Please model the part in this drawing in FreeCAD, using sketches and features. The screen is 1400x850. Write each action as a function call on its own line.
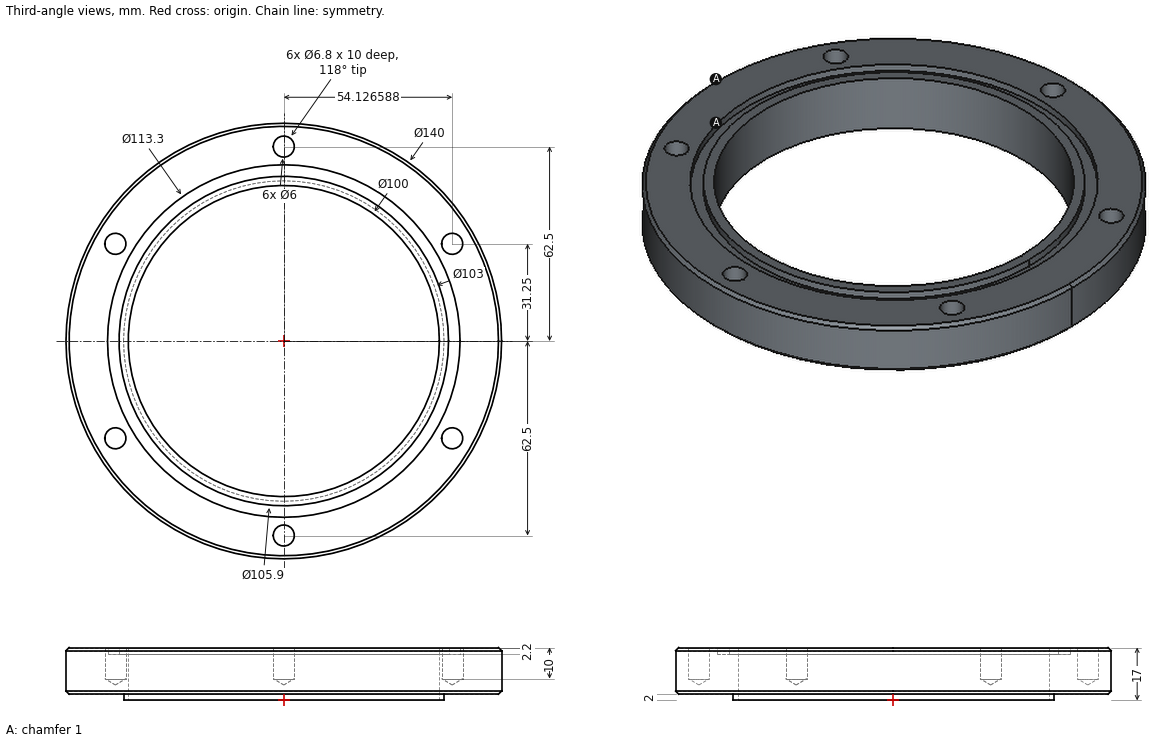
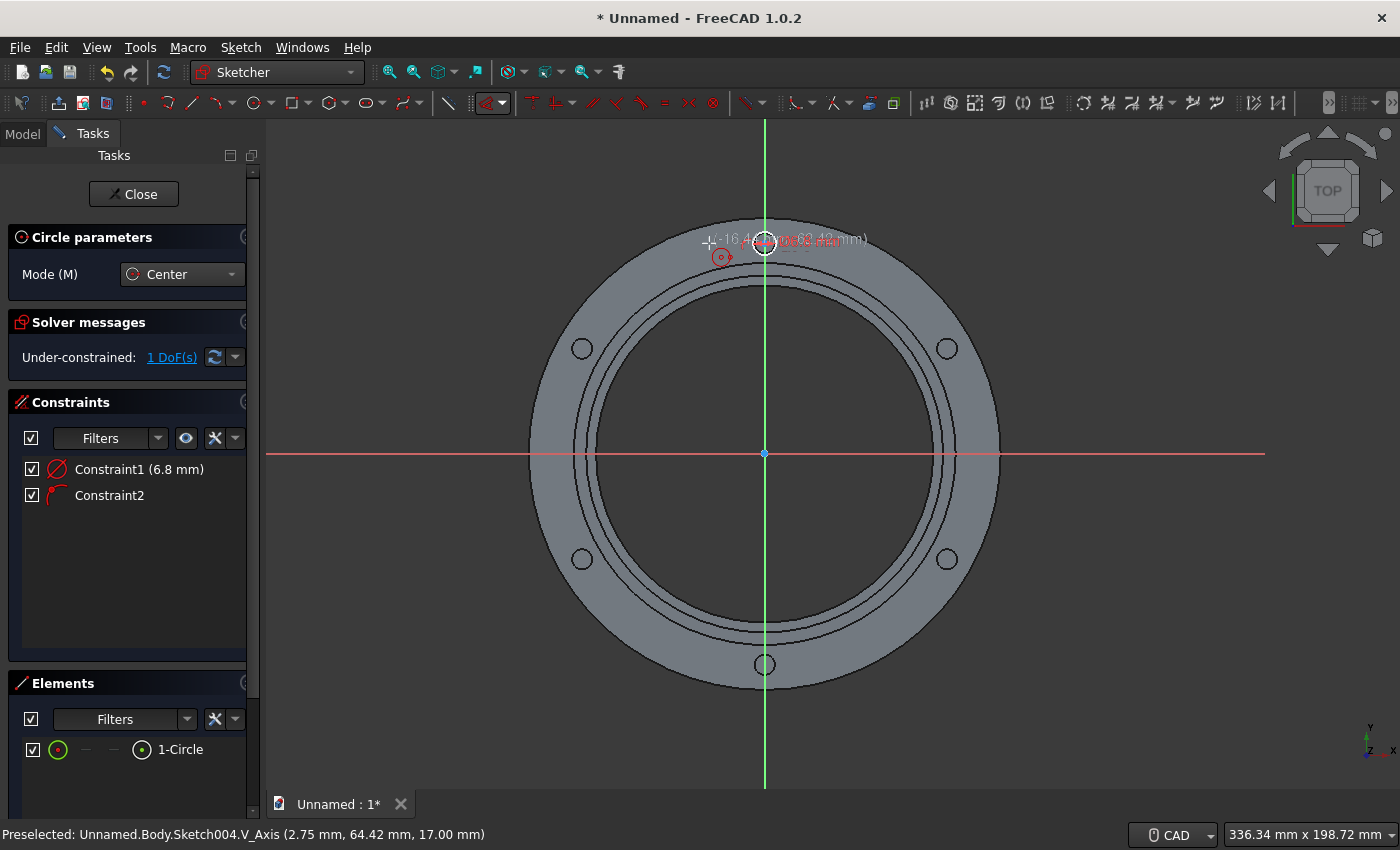
scroll(947, 349, up, 4)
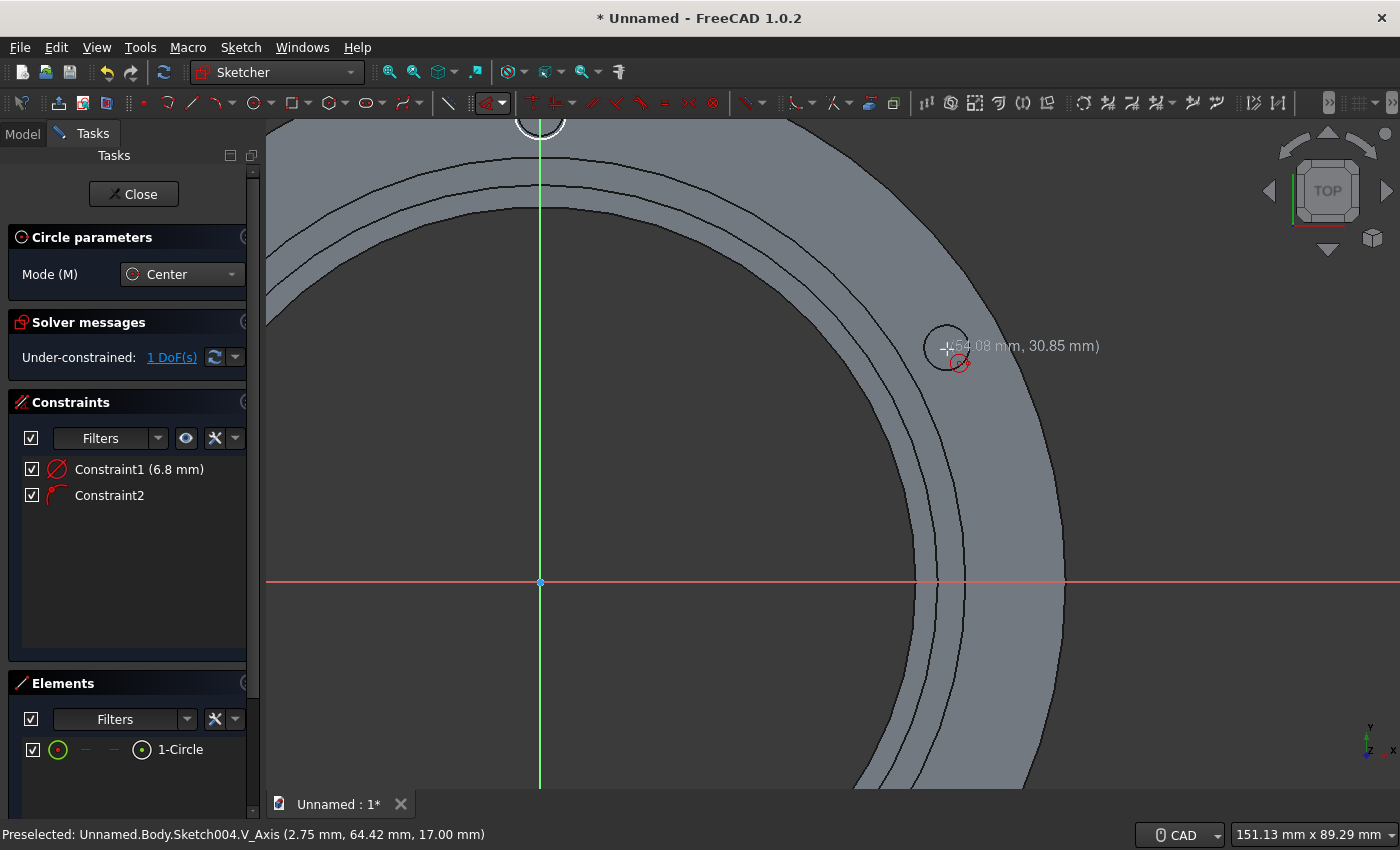
click(947, 348)
move(965, 330)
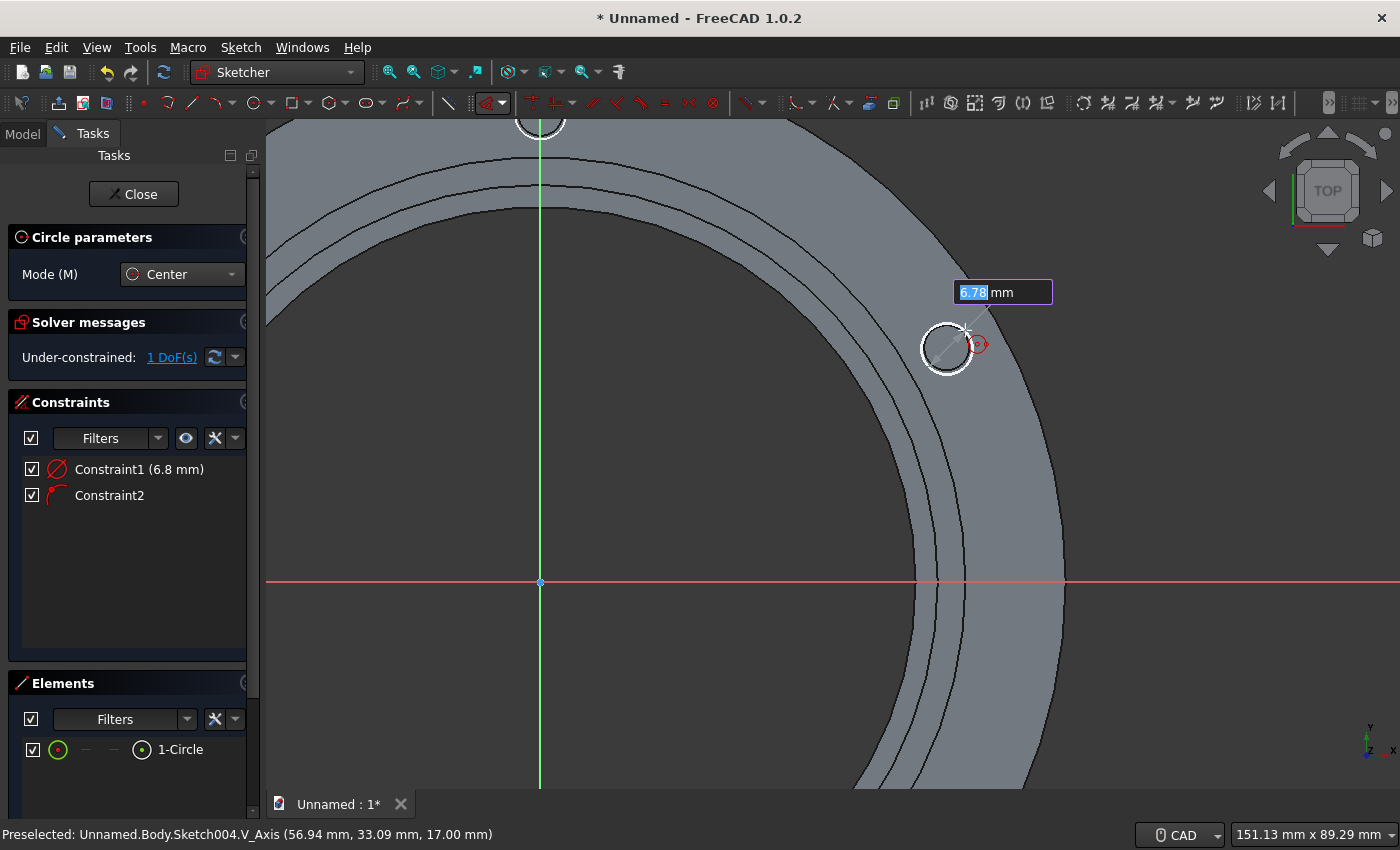
text(6.8)
key(Return)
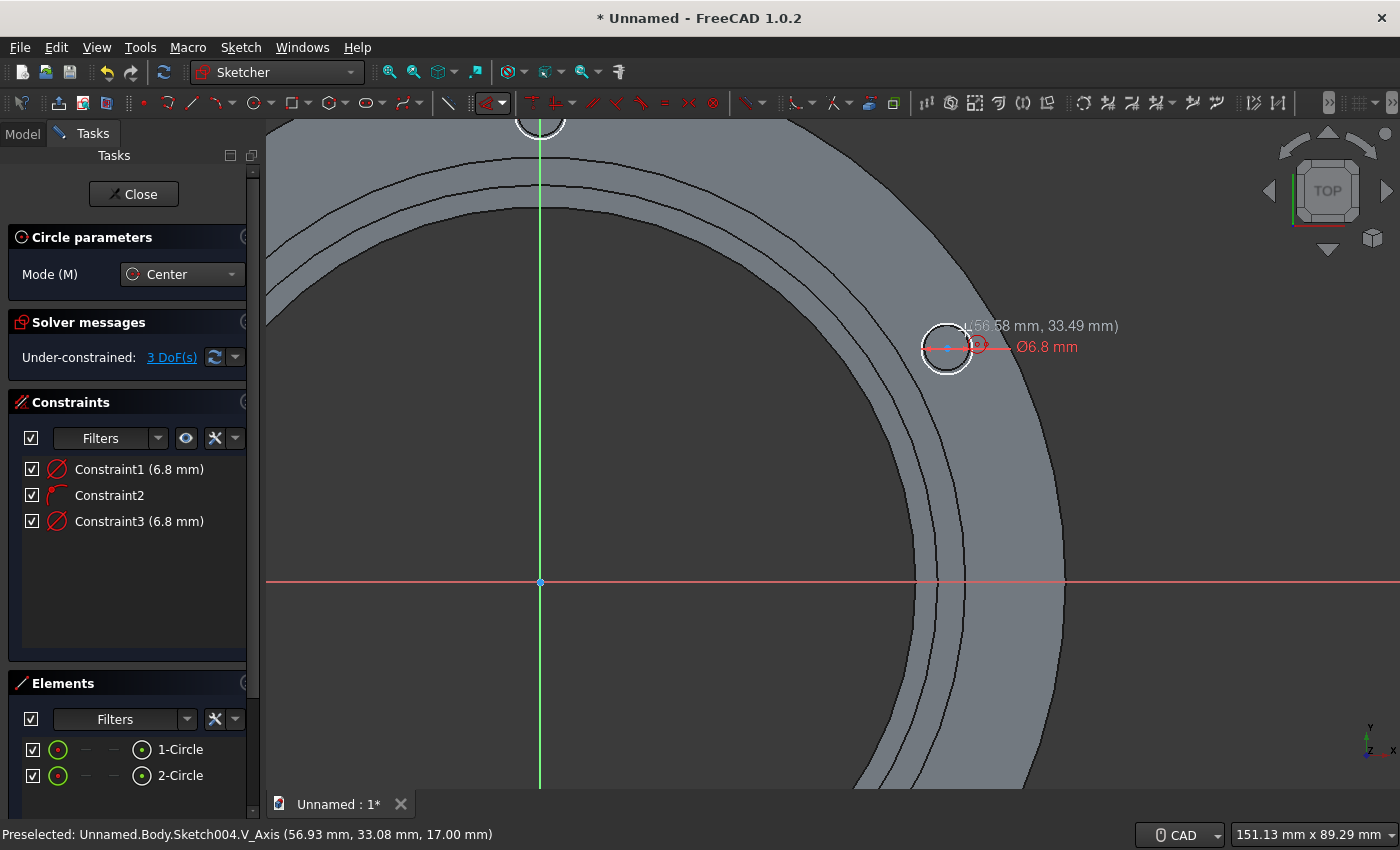
scroll(947, 349, down, 4)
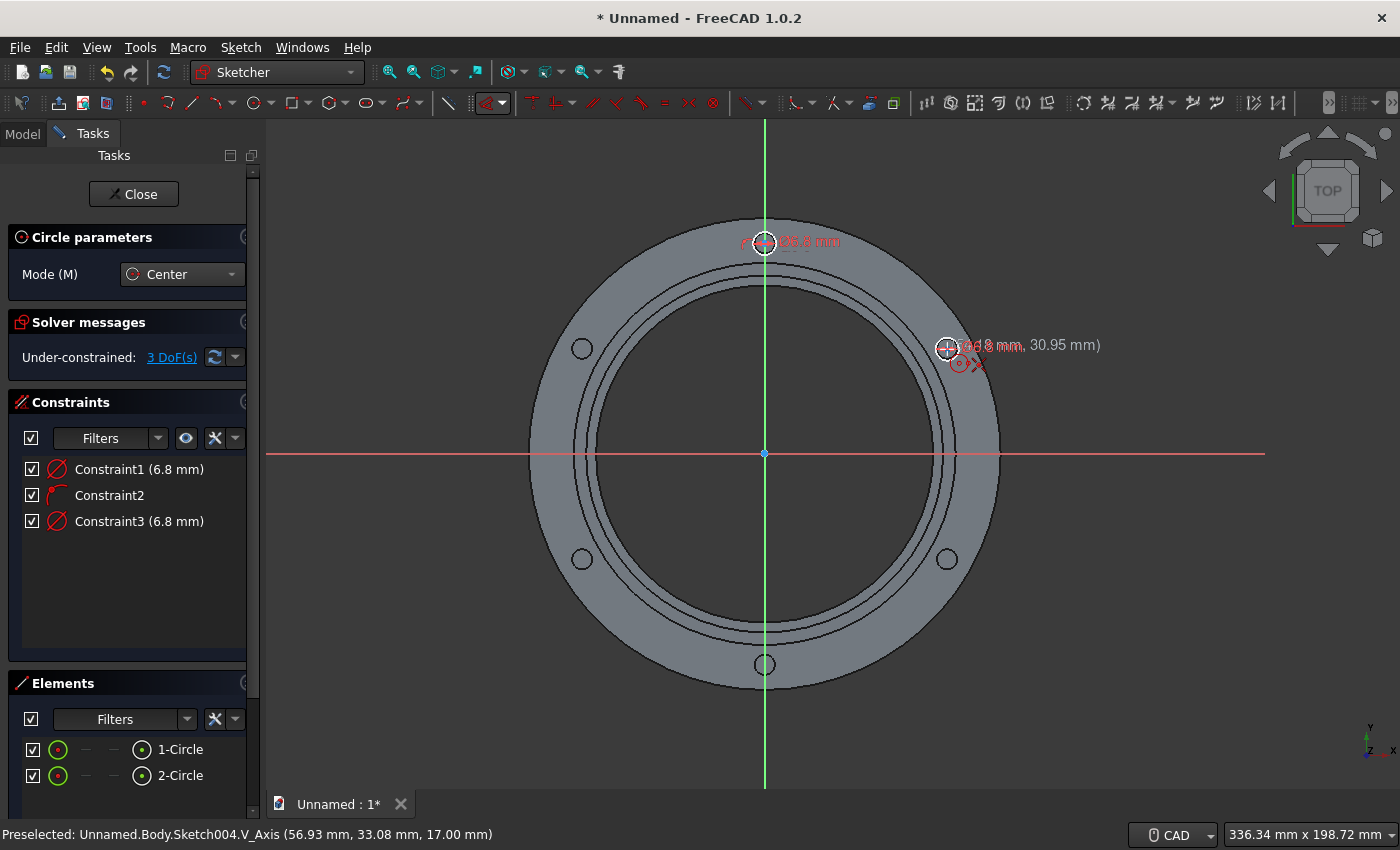
scroll(947, 559, up, 4)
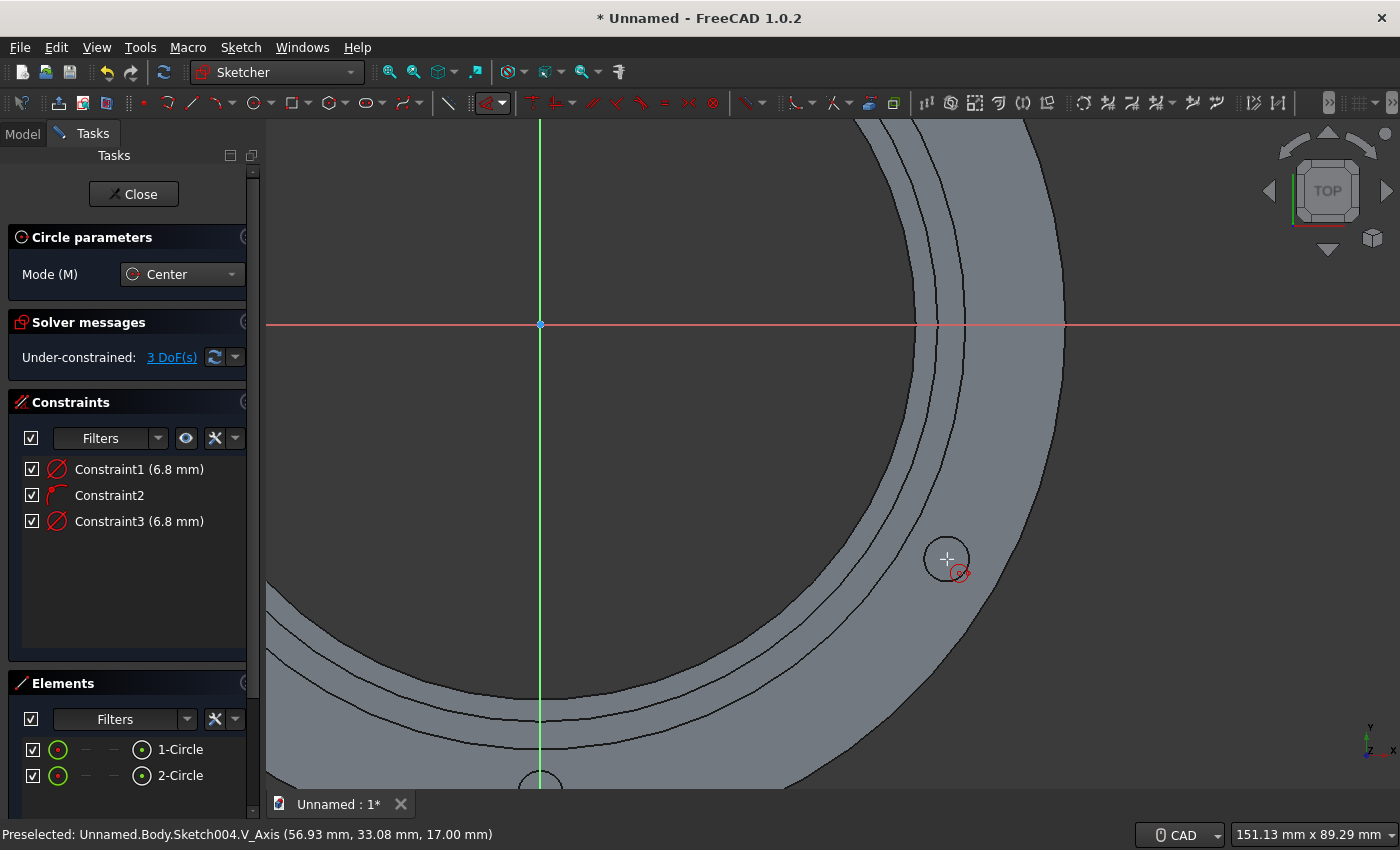
click(947, 559)
move(965, 541)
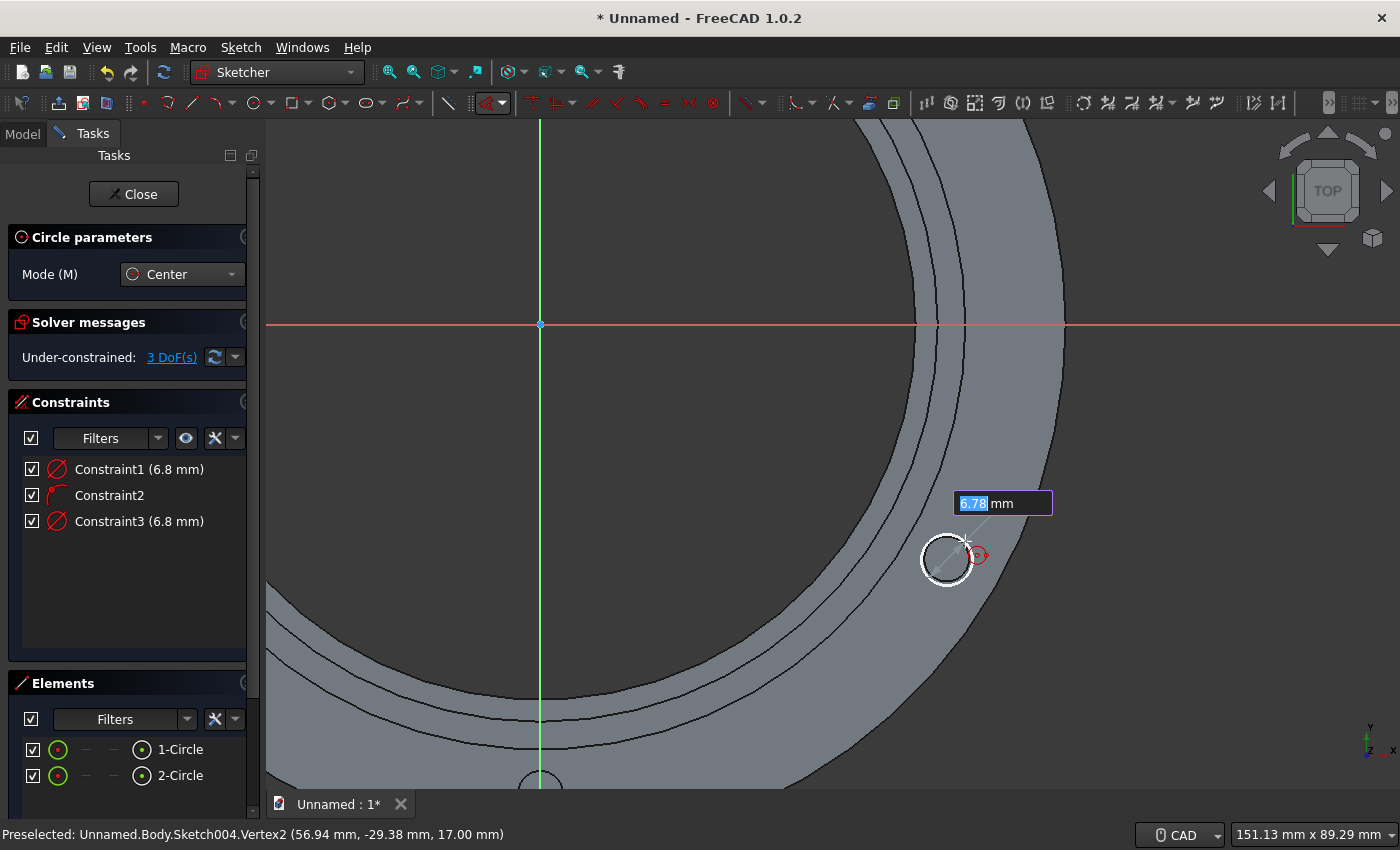
text(6.8)
key(Return)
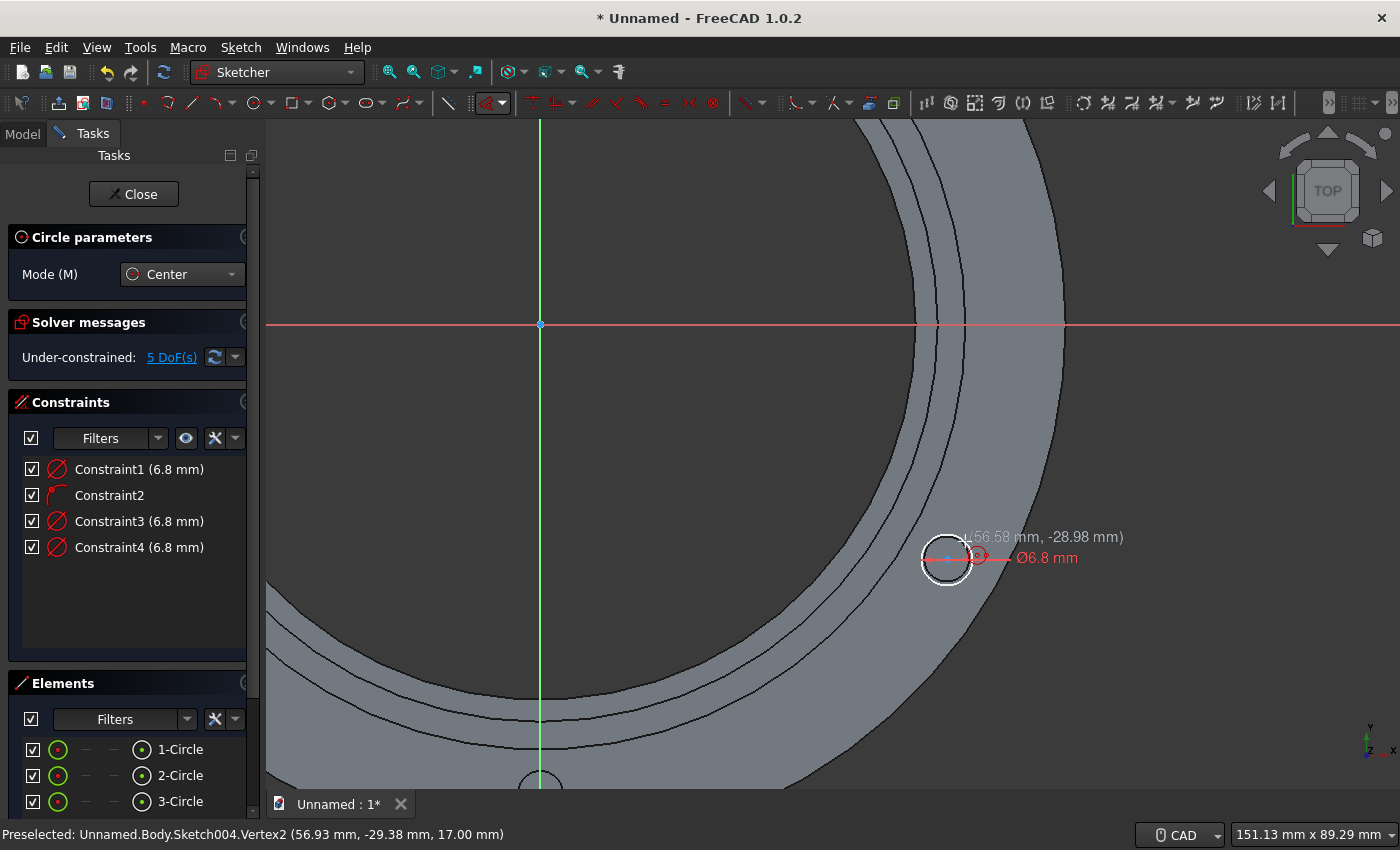
scroll(947, 560, down, 4)